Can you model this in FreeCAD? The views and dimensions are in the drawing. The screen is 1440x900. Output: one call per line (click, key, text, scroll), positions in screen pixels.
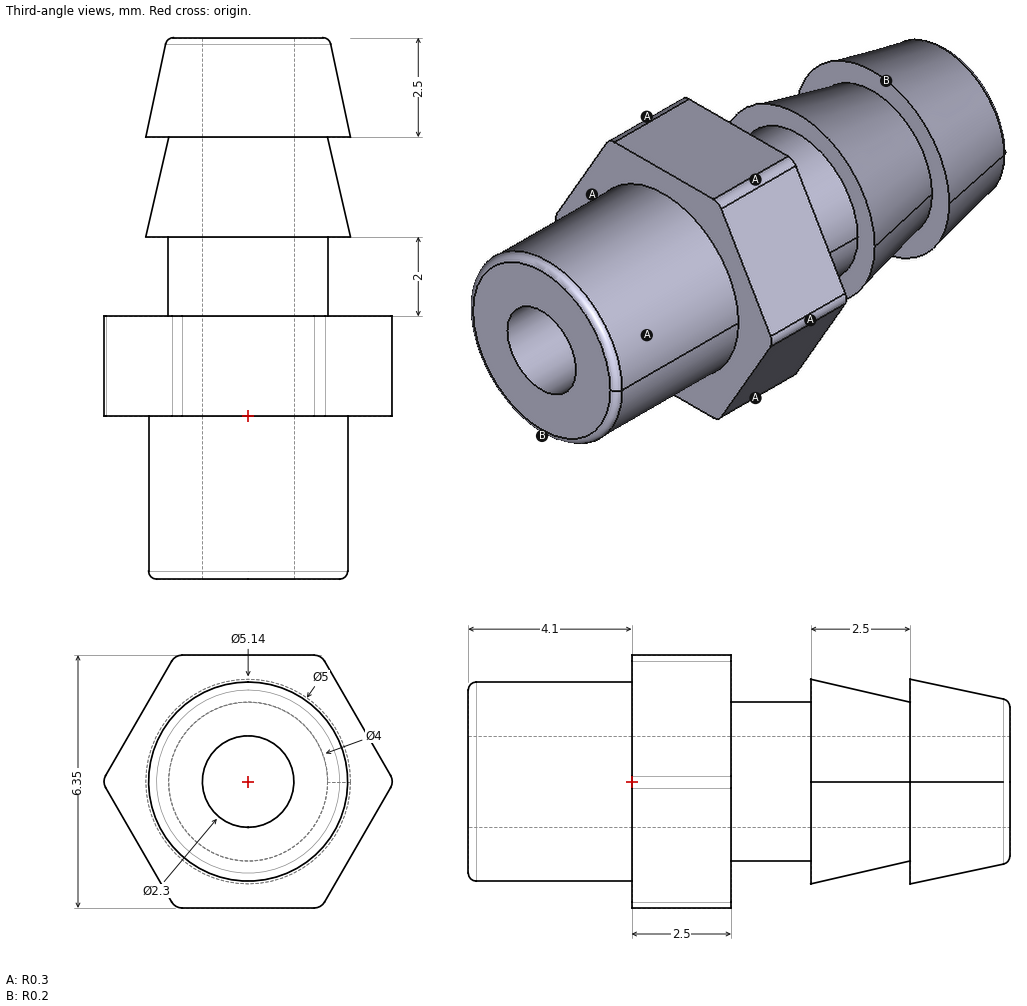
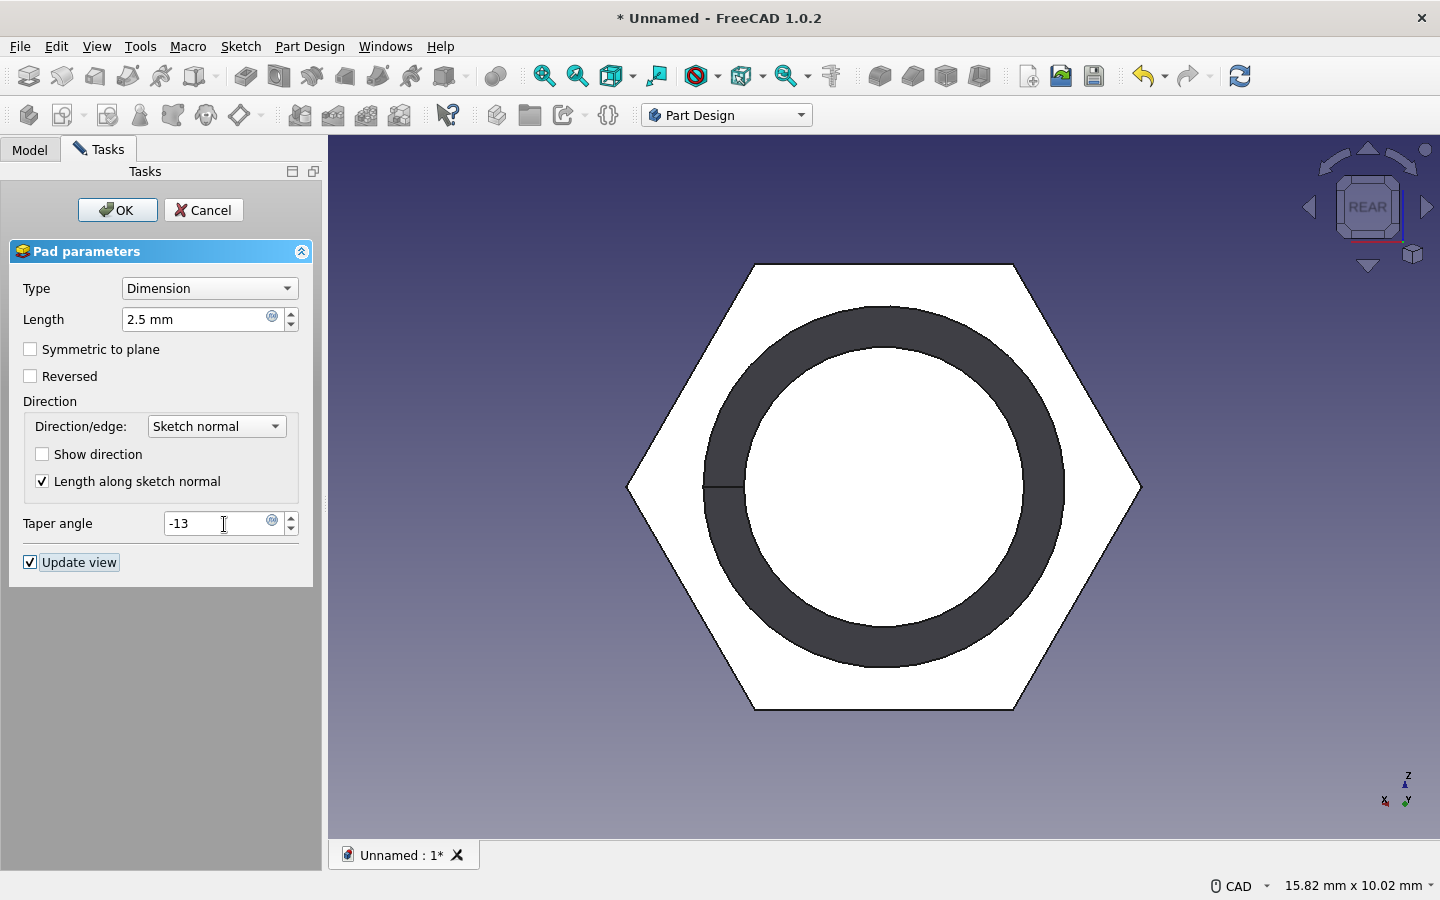
click(118, 210)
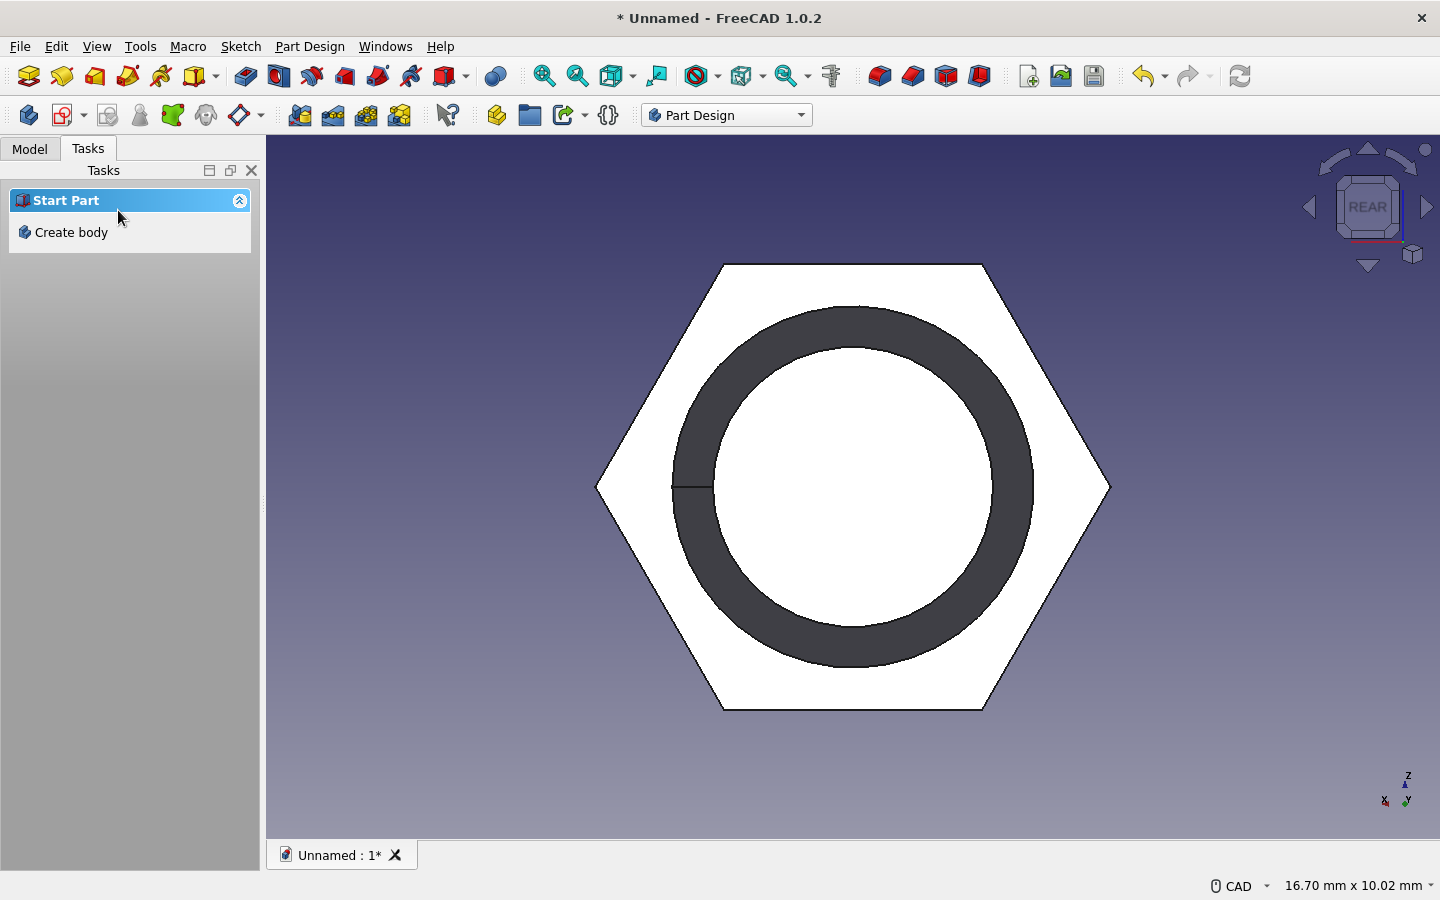
click(853, 486)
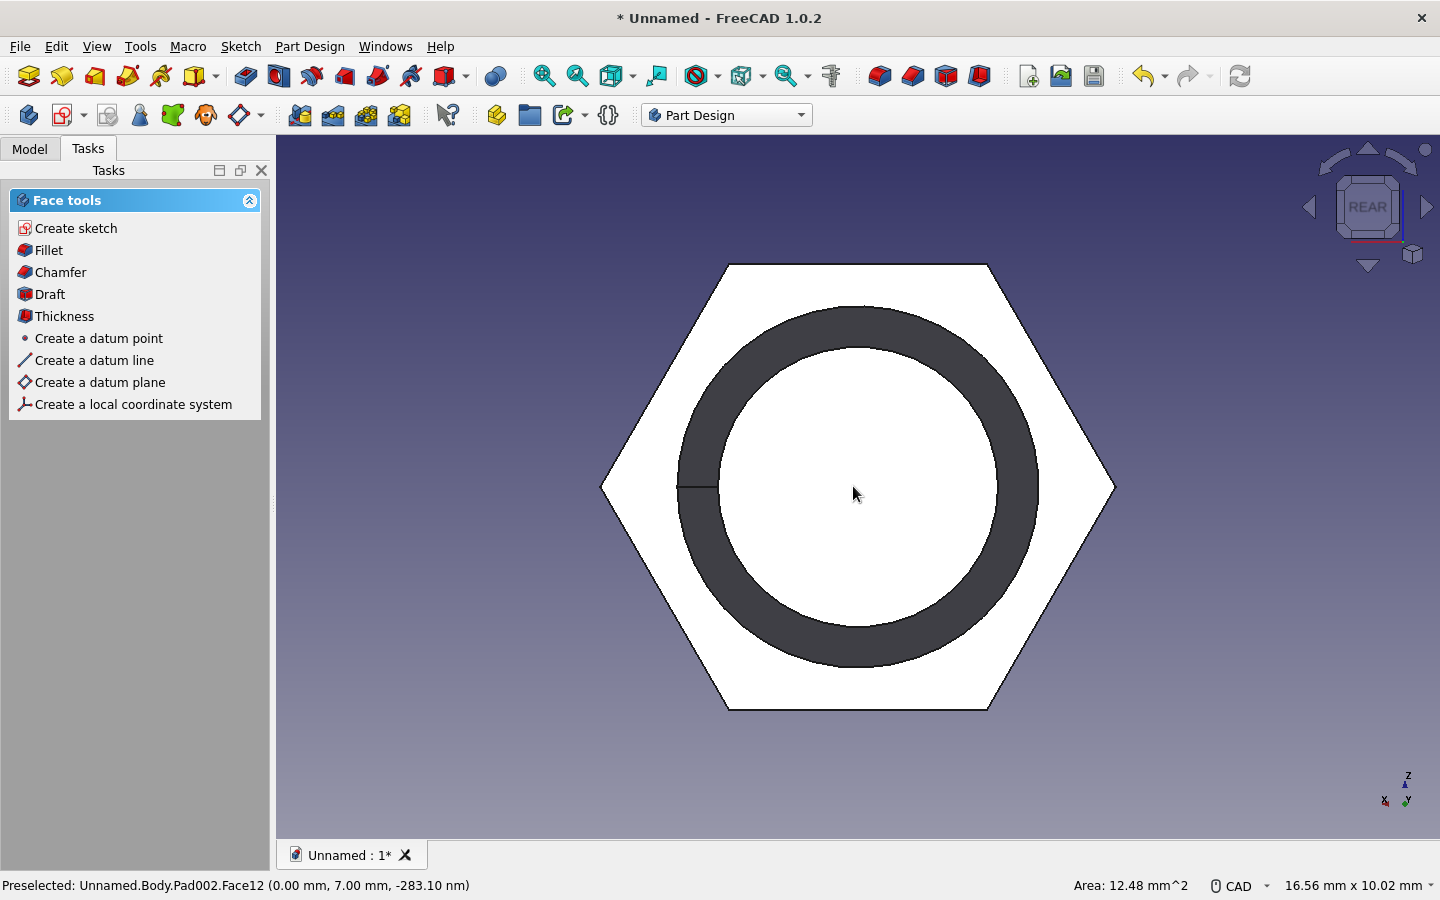
click(62, 116)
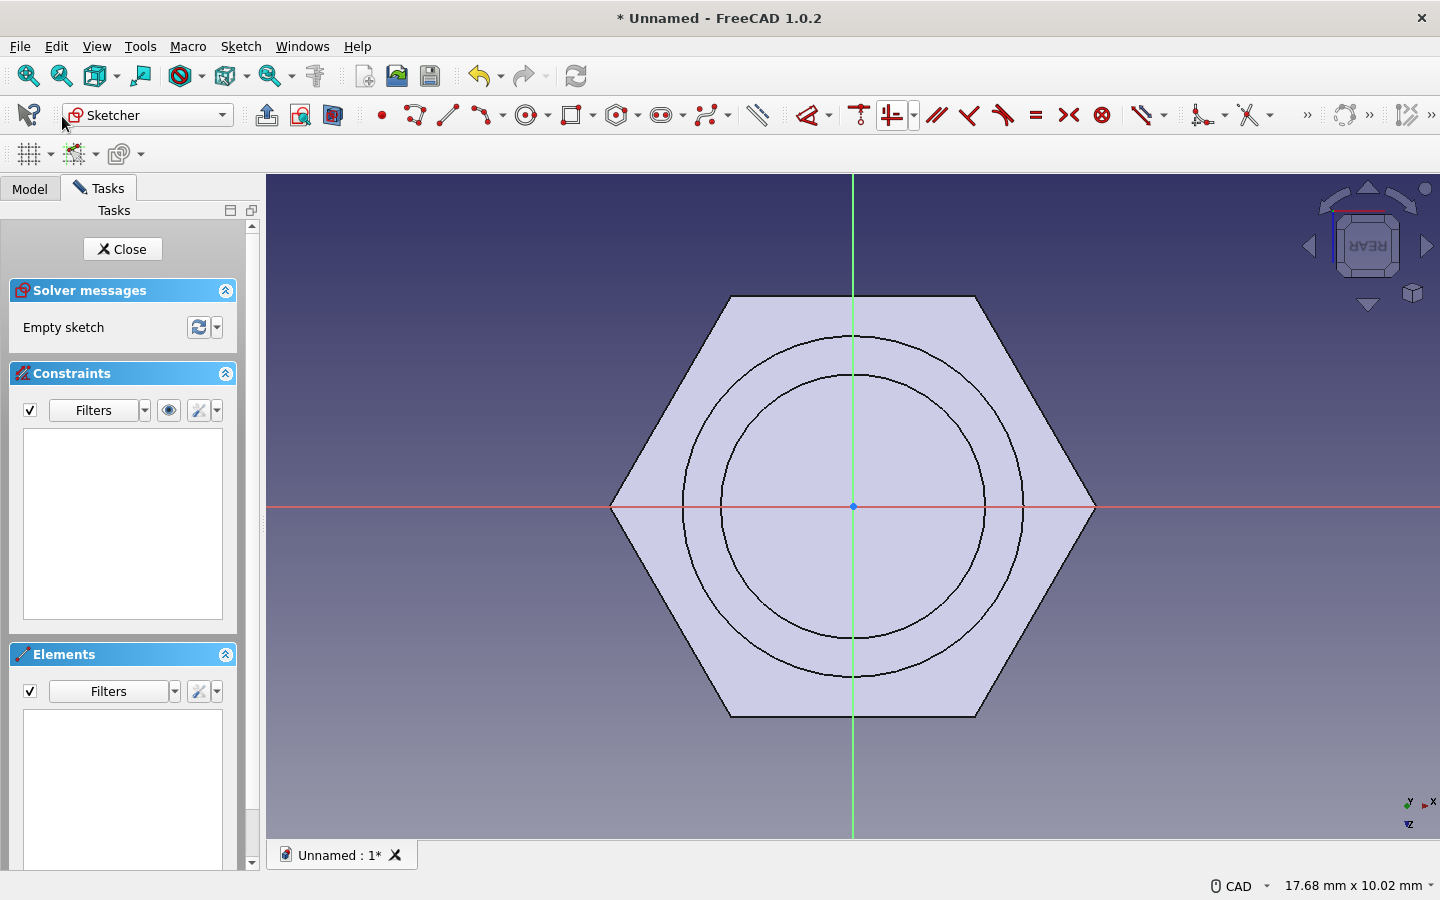
key(g)
key(c)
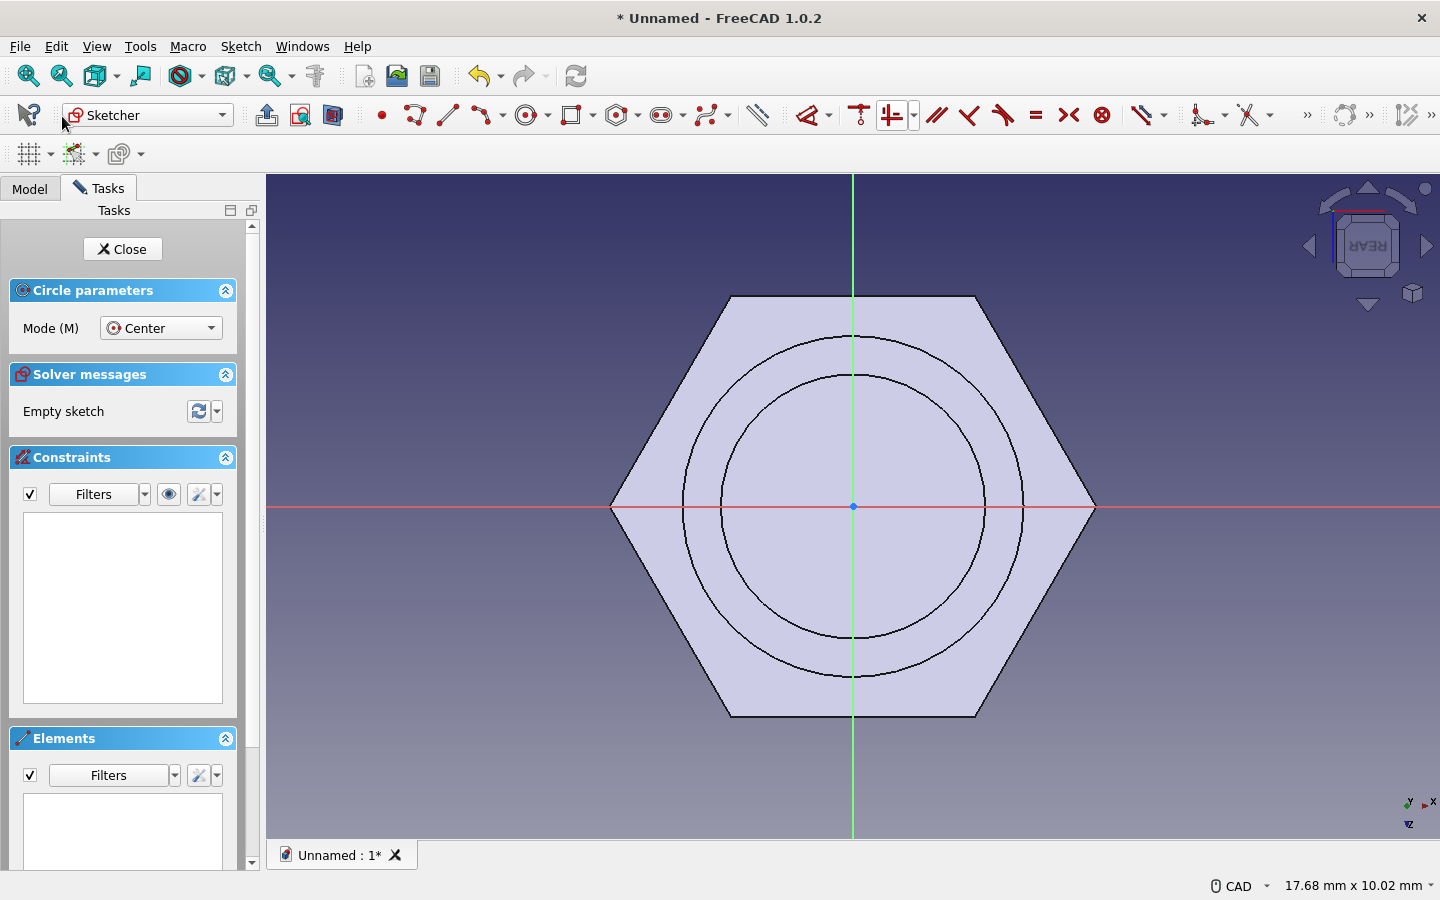
click(853, 507)
click(974, 386)
key(Escape)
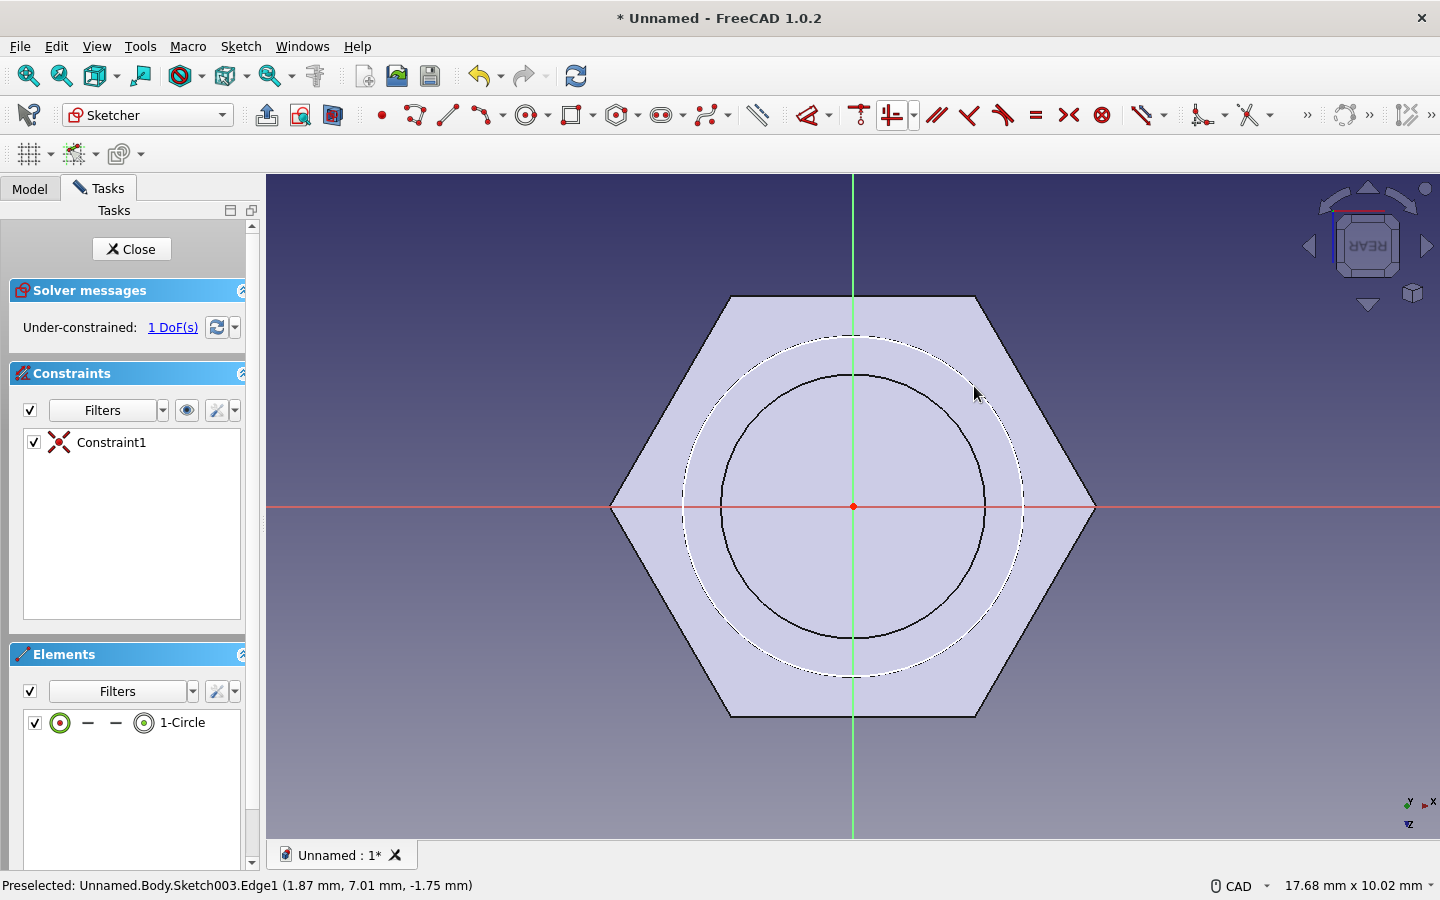
click(806, 116)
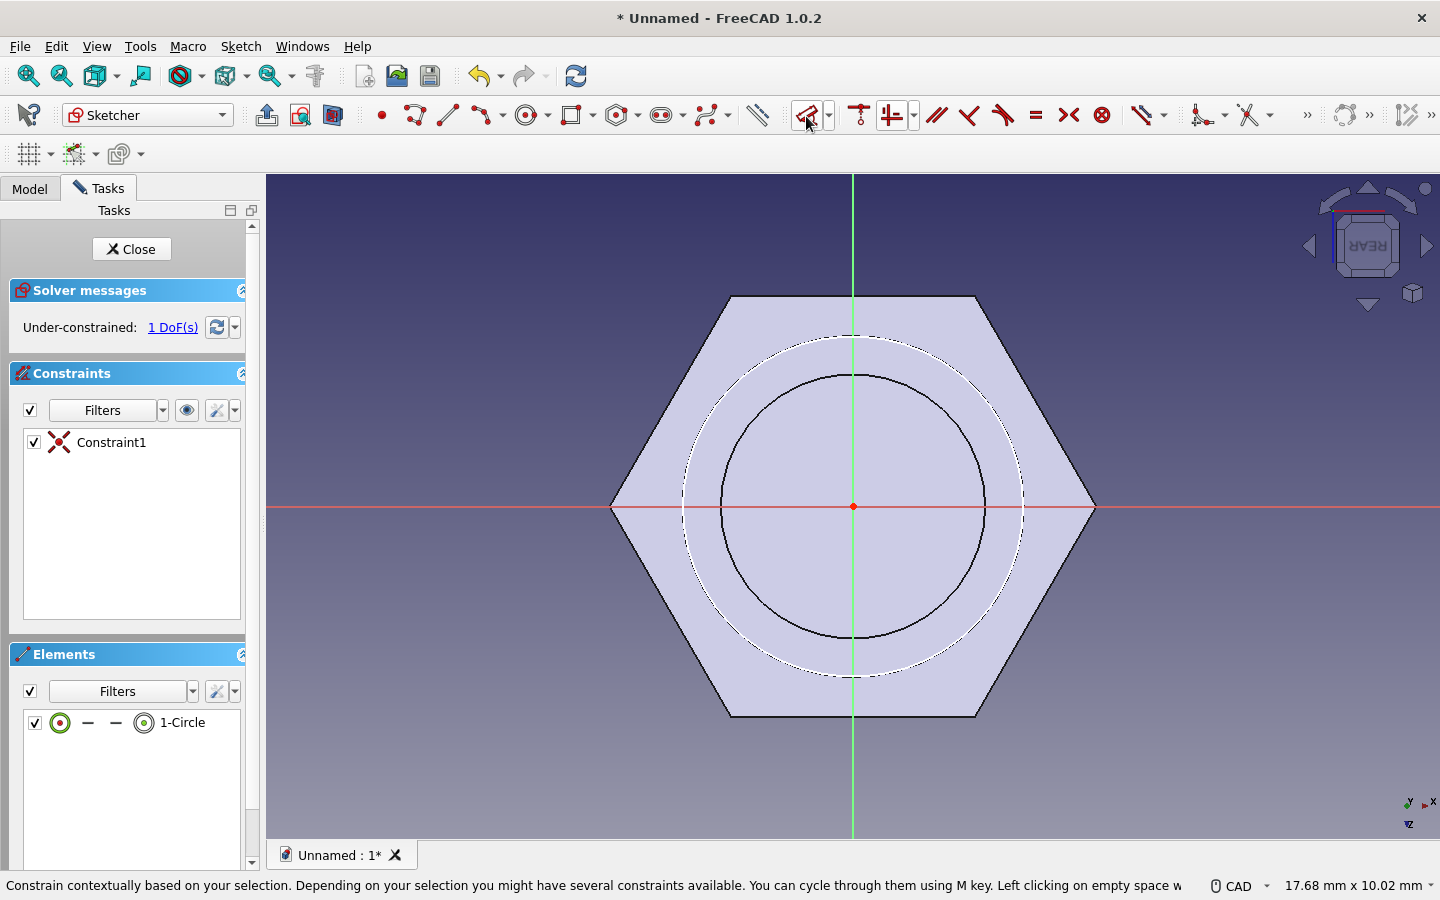
click(973, 386)
click(996, 363)